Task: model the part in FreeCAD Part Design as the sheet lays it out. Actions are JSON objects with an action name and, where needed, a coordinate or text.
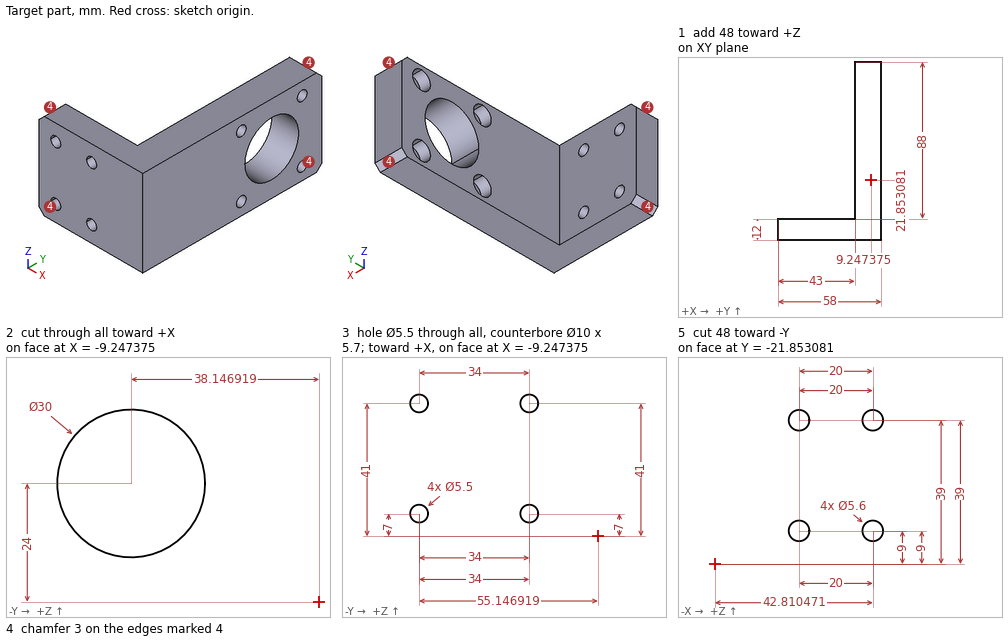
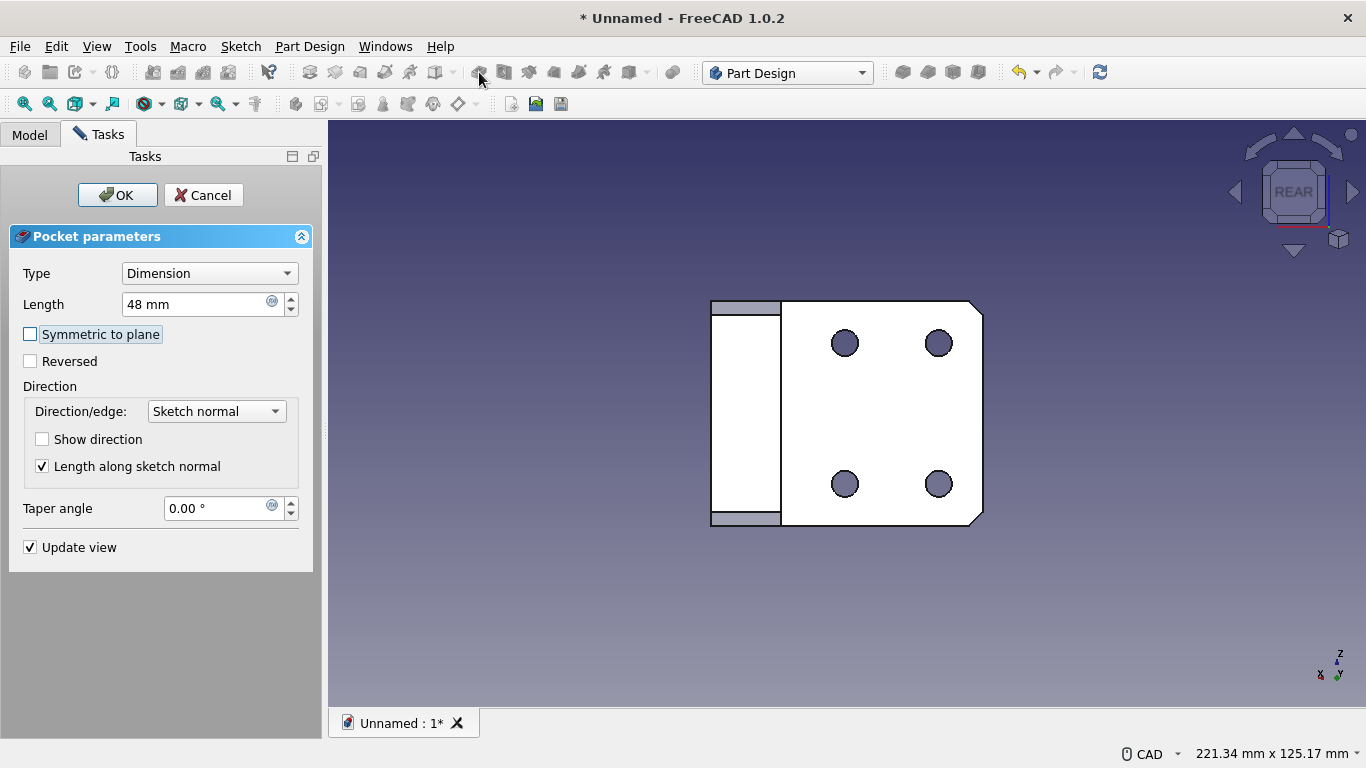
{"action": "left_click", "coordinate": [118, 195]}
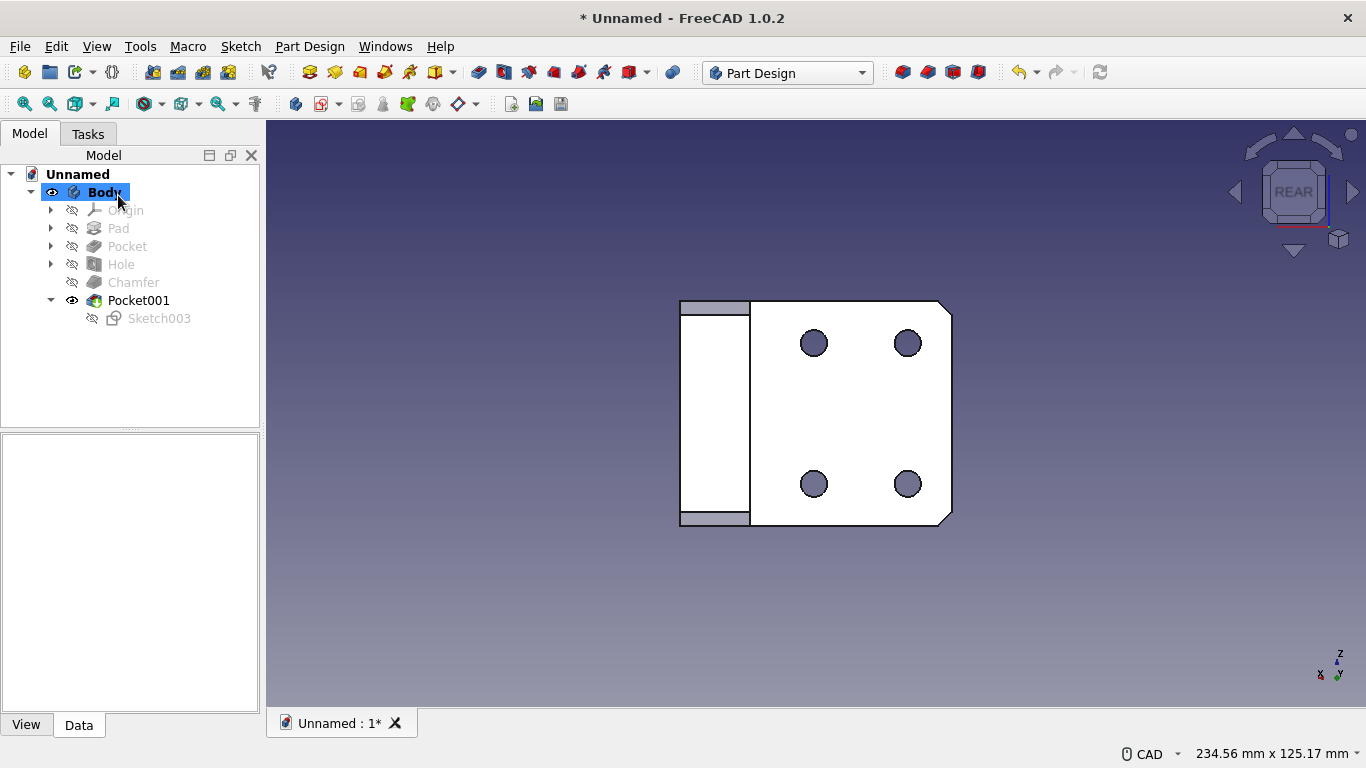
{"action": "key", "text": "0"}